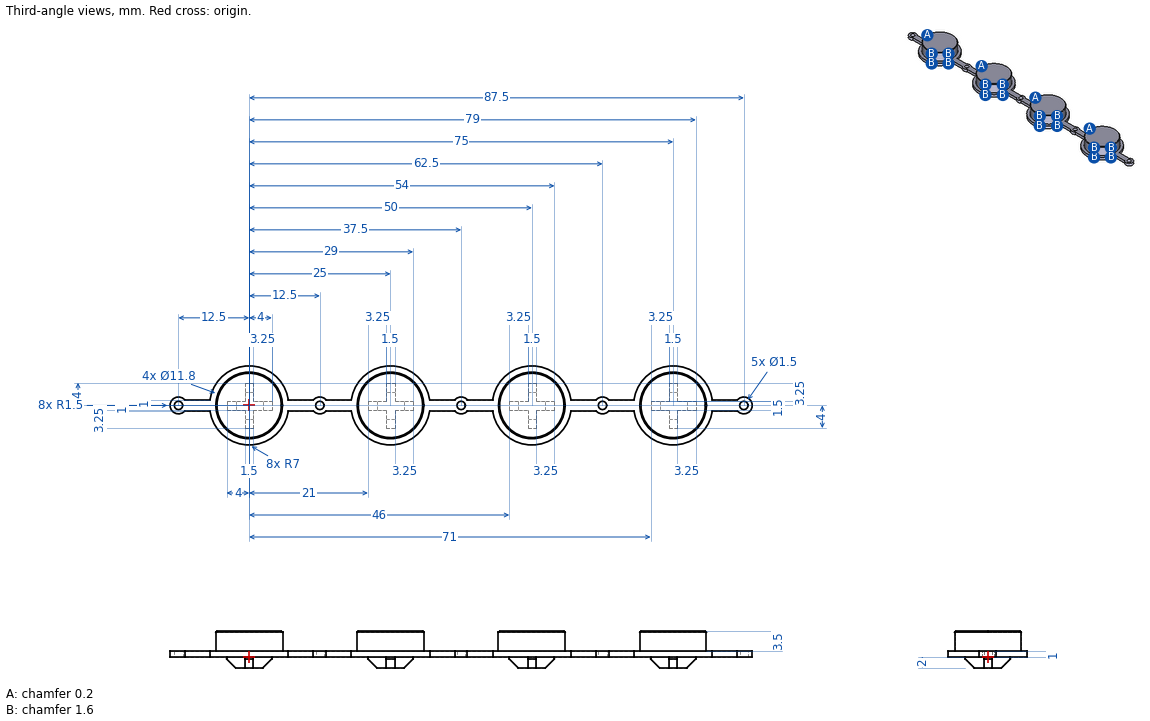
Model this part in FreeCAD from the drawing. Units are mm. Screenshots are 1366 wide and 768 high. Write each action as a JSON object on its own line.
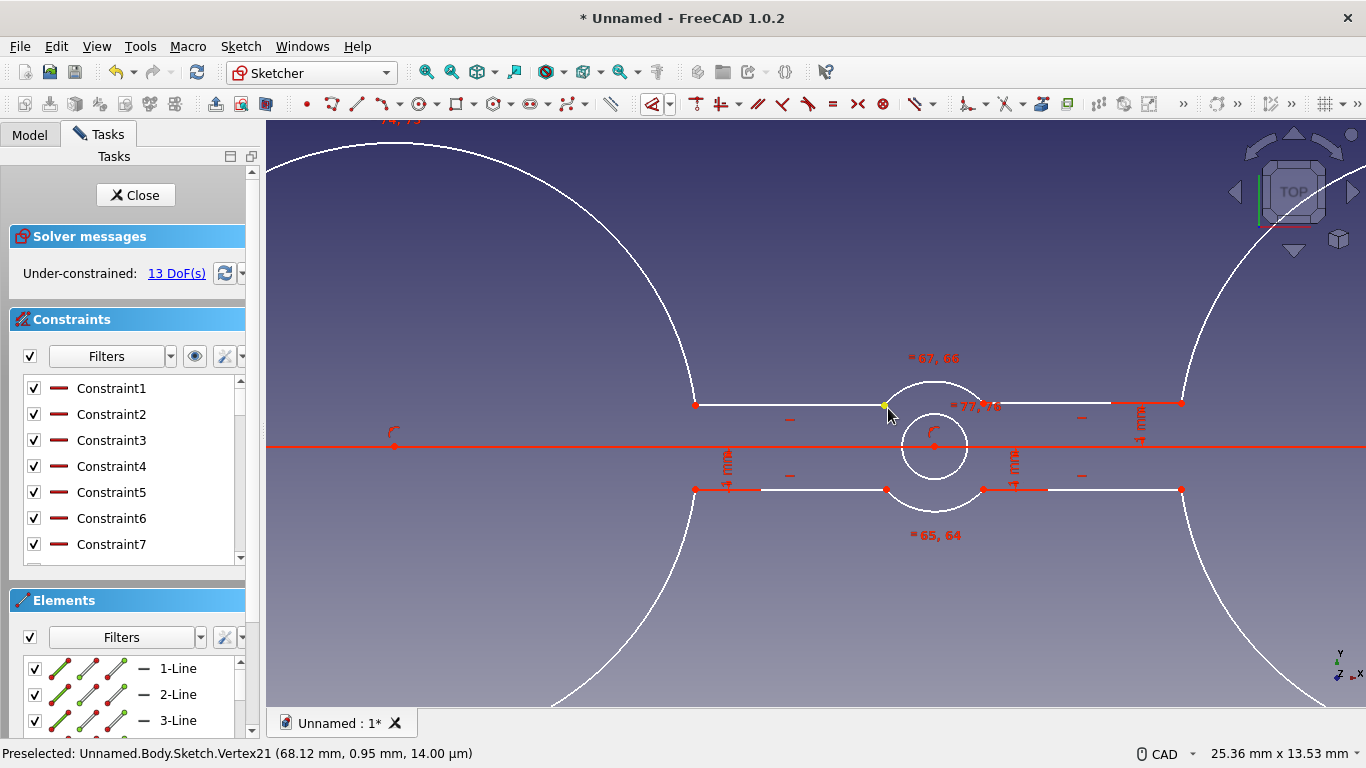
{"action": "left_click", "coordinate": [884, 405]}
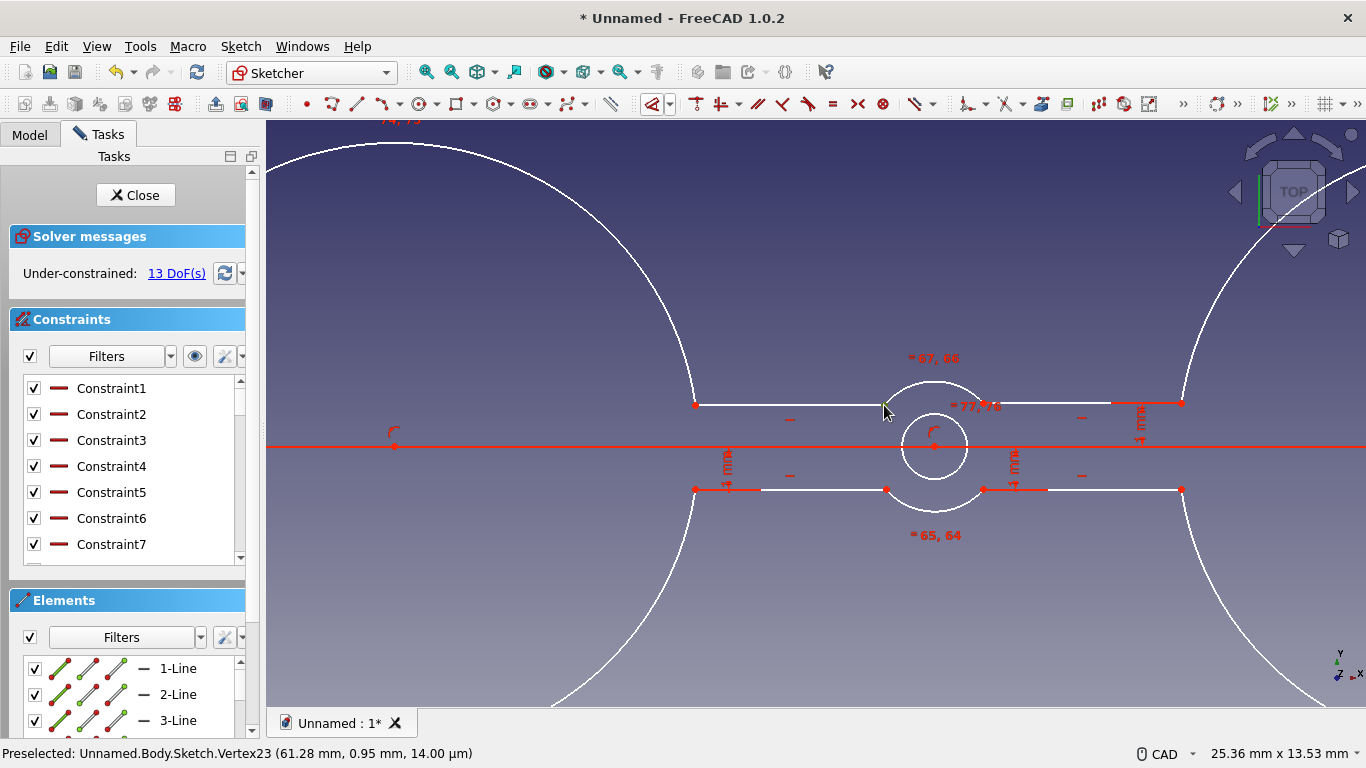
{"action": "key", "text": "i"}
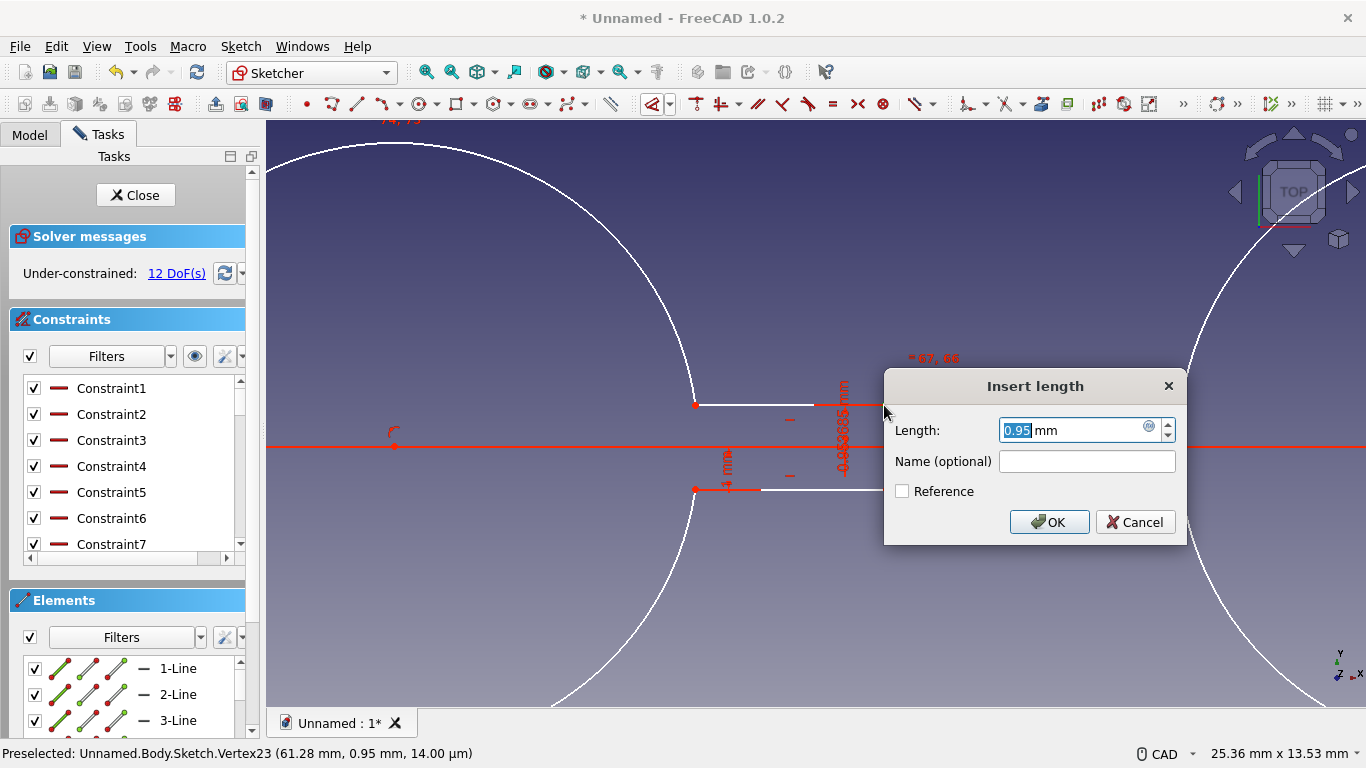
{"action": "type", "text": "1"}
{"action": "key", "text": "Return"}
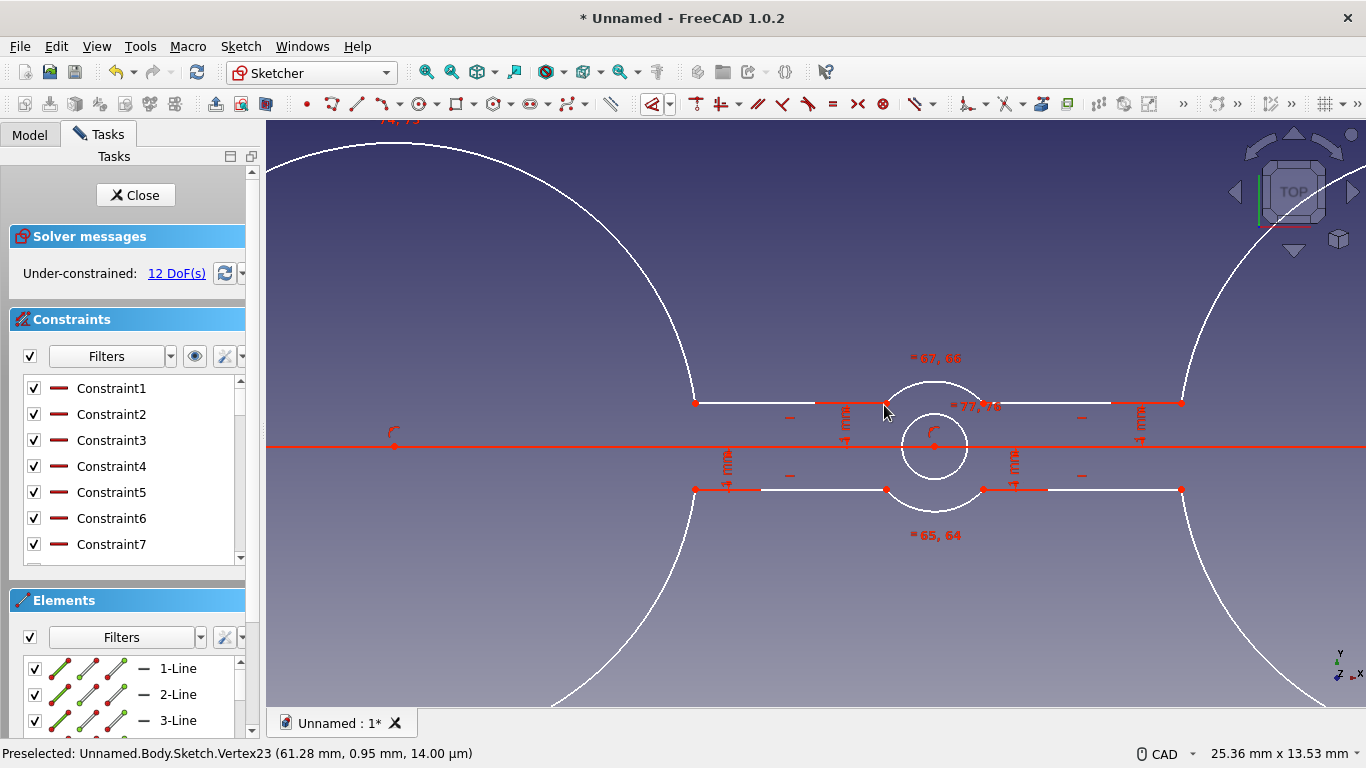
{"action": "scroll", "coordinate": [887, 408], "scroll_direction": "down", "scroll_amount": 10}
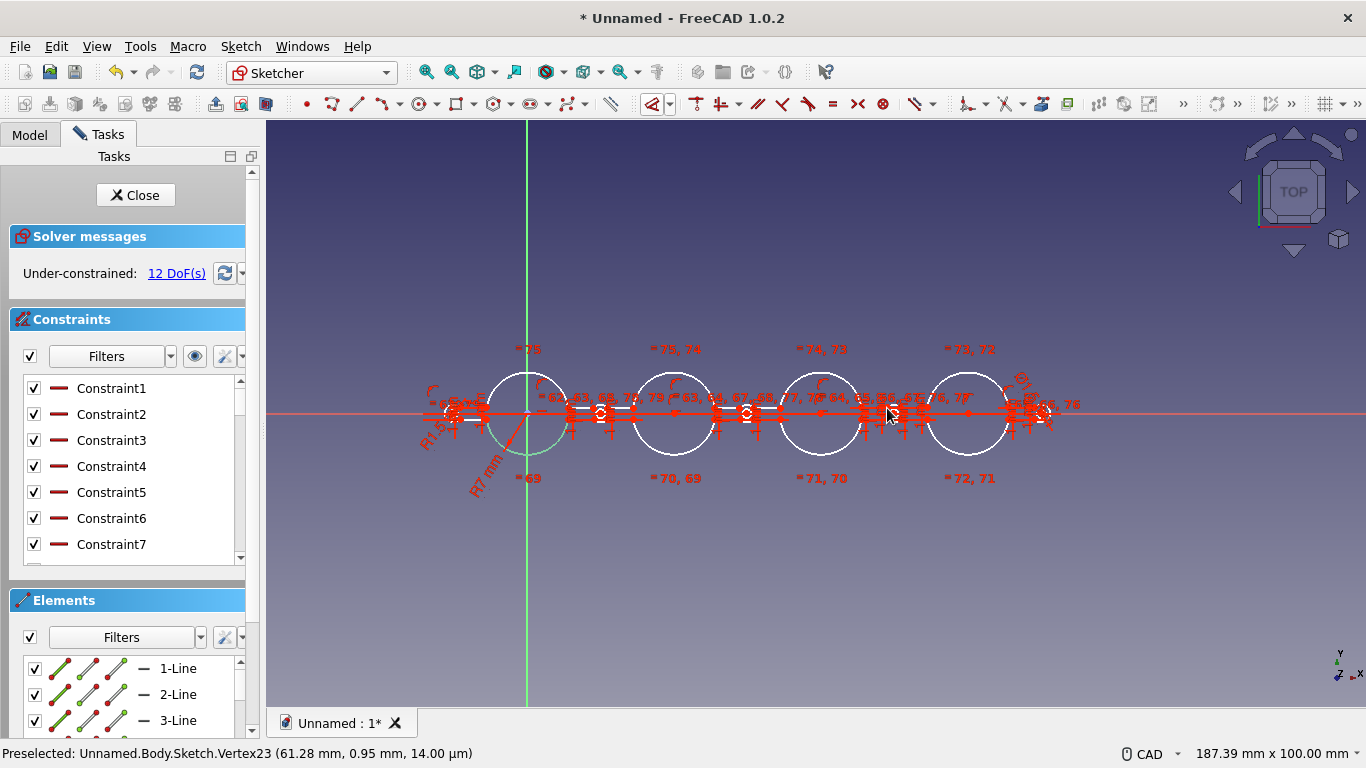
{"action": "scroll", "coordinate": [780, 408], "scroll_direction": "up", "scroll_amount": 10}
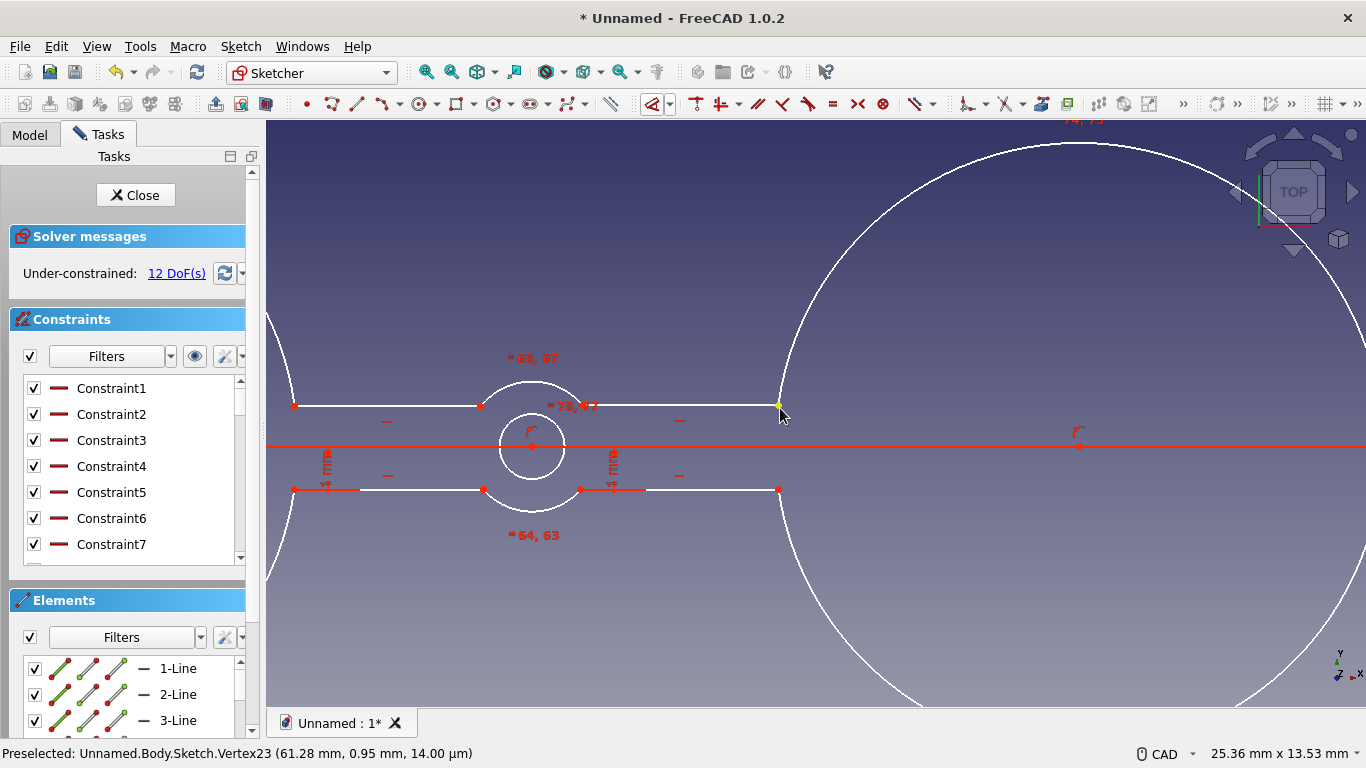
{"action": "left_click", "coordinate": [778, 405]}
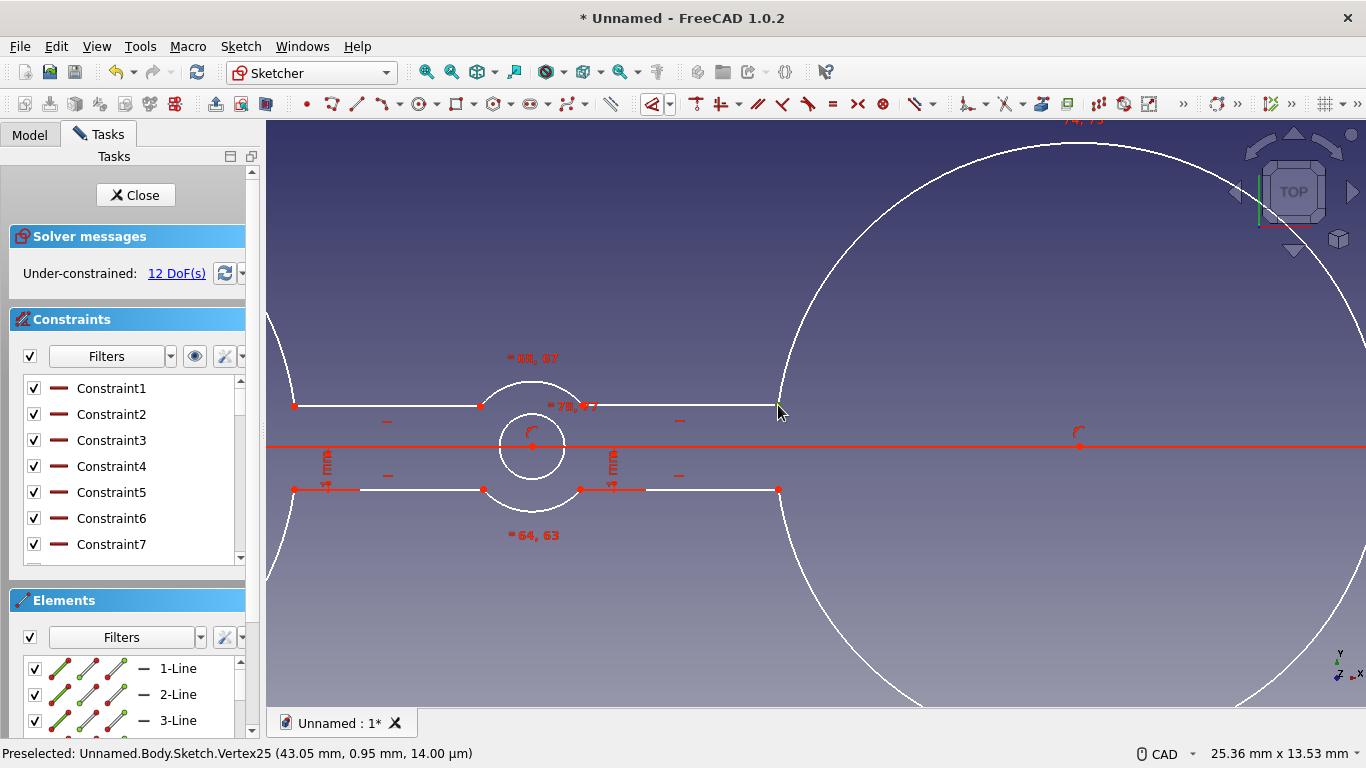
{"action": "key", "text": "i"}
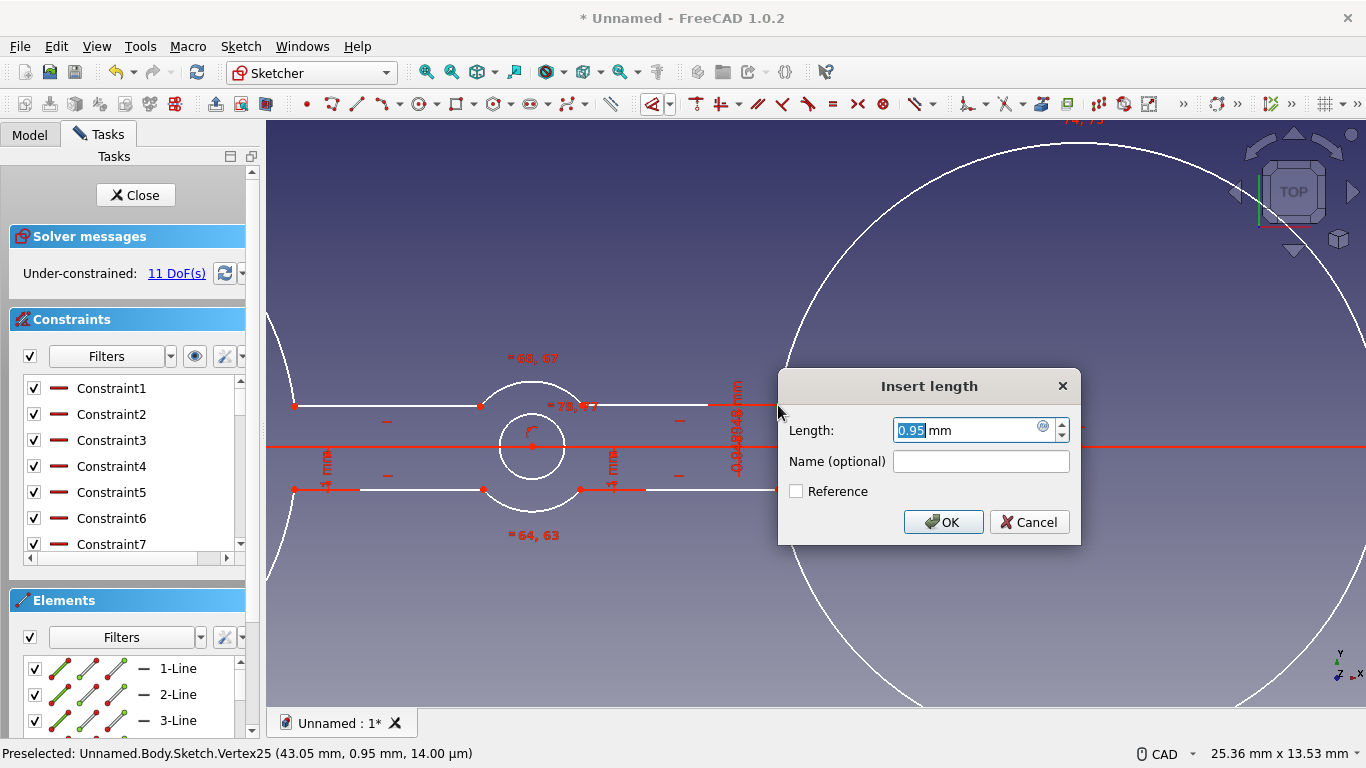
{"action": "type", "text": "1"}
{"action": "key", "text": "Return"}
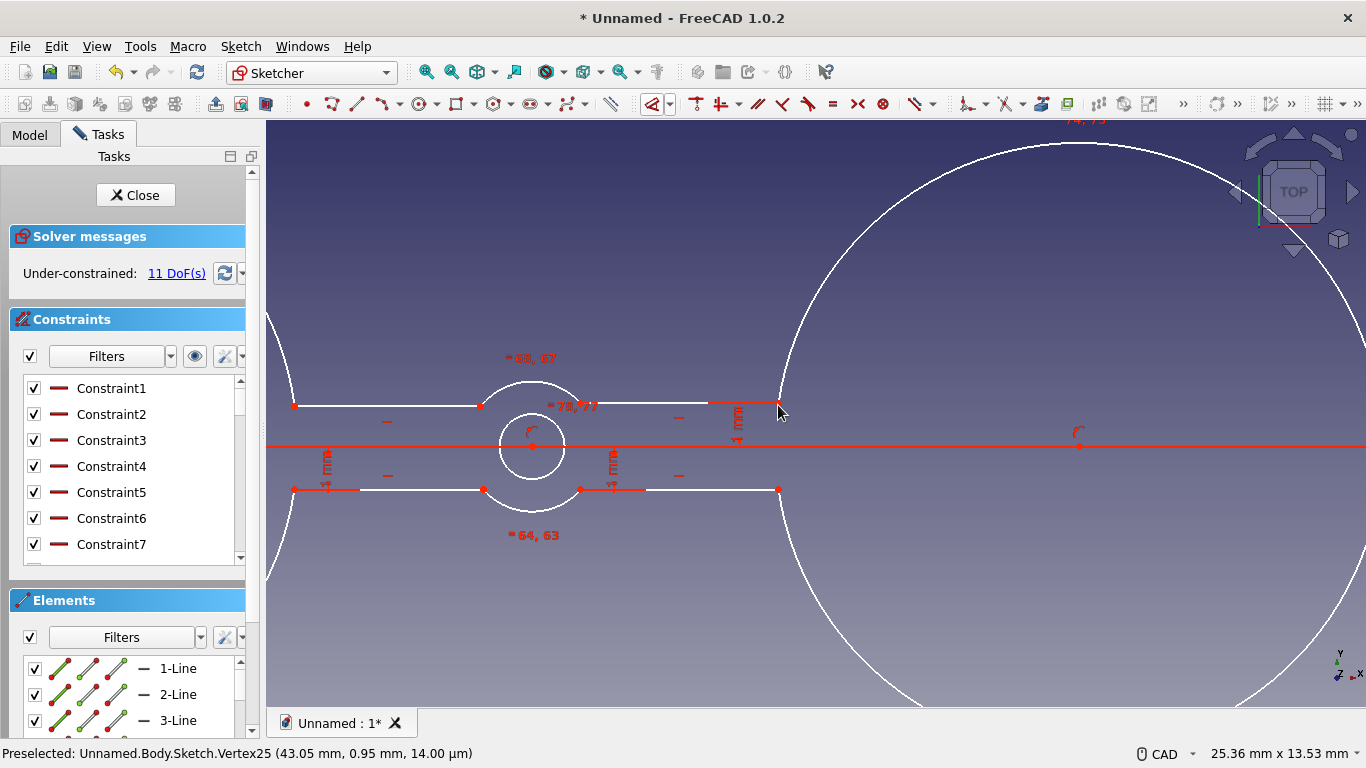
{"action": "left_click", "coordinate": [481, 406]}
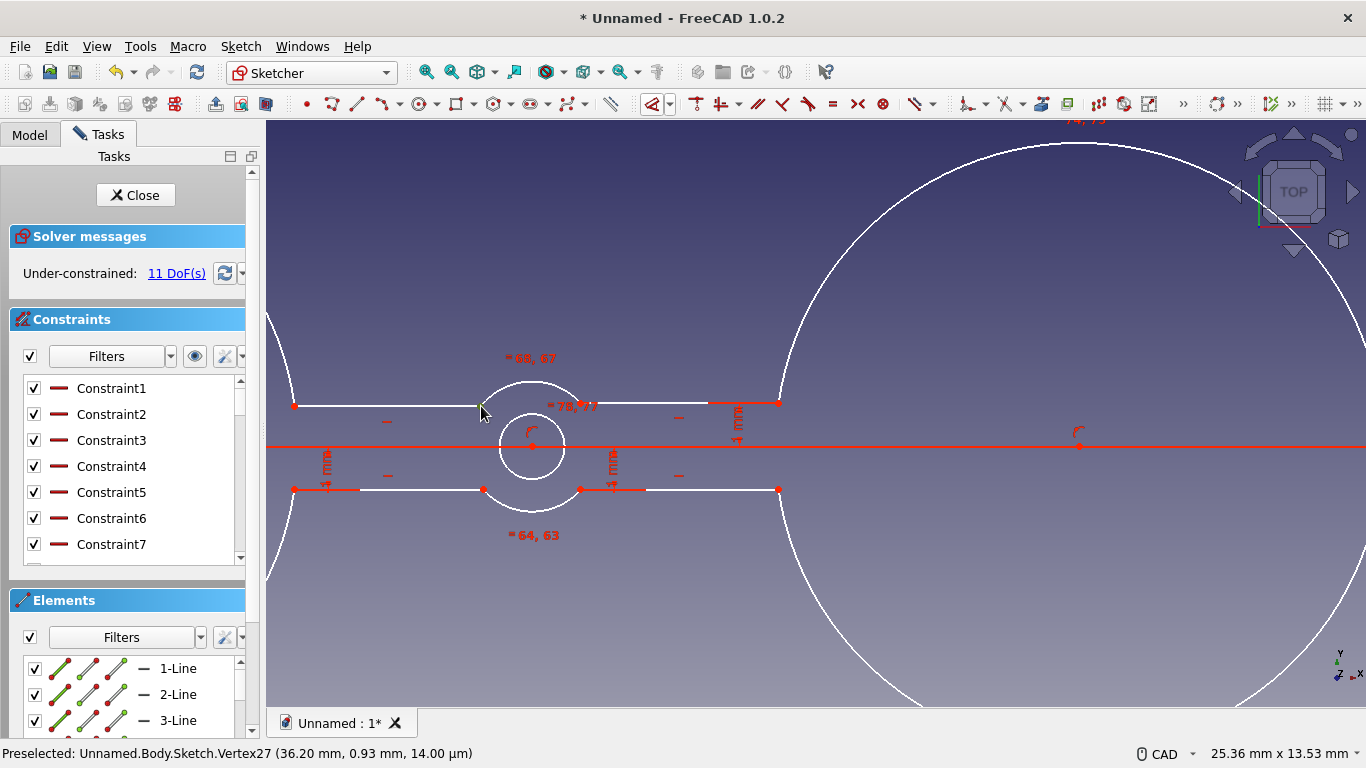
{"action": "key", "text": "i"}